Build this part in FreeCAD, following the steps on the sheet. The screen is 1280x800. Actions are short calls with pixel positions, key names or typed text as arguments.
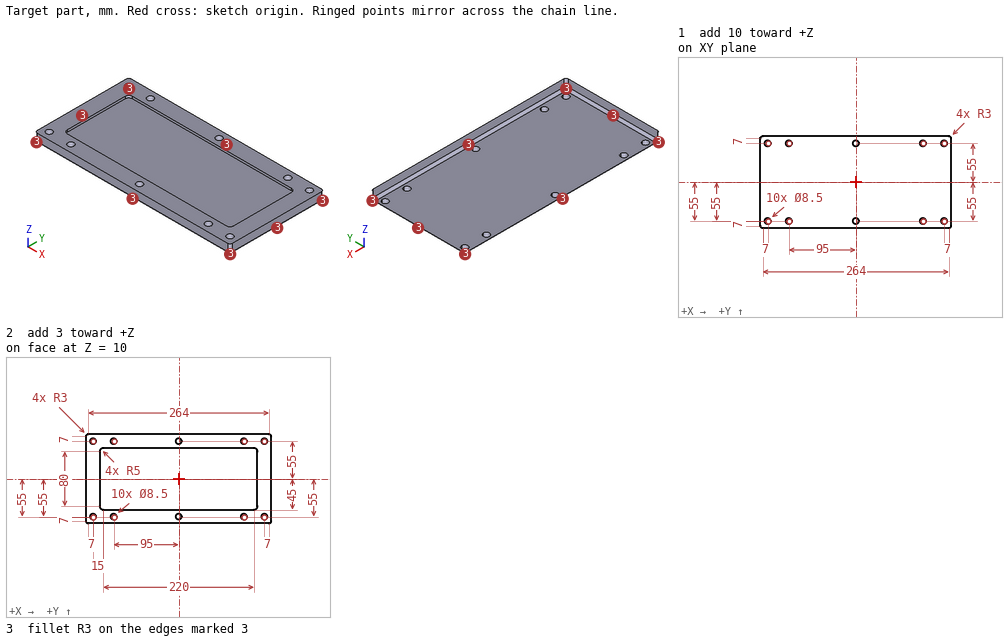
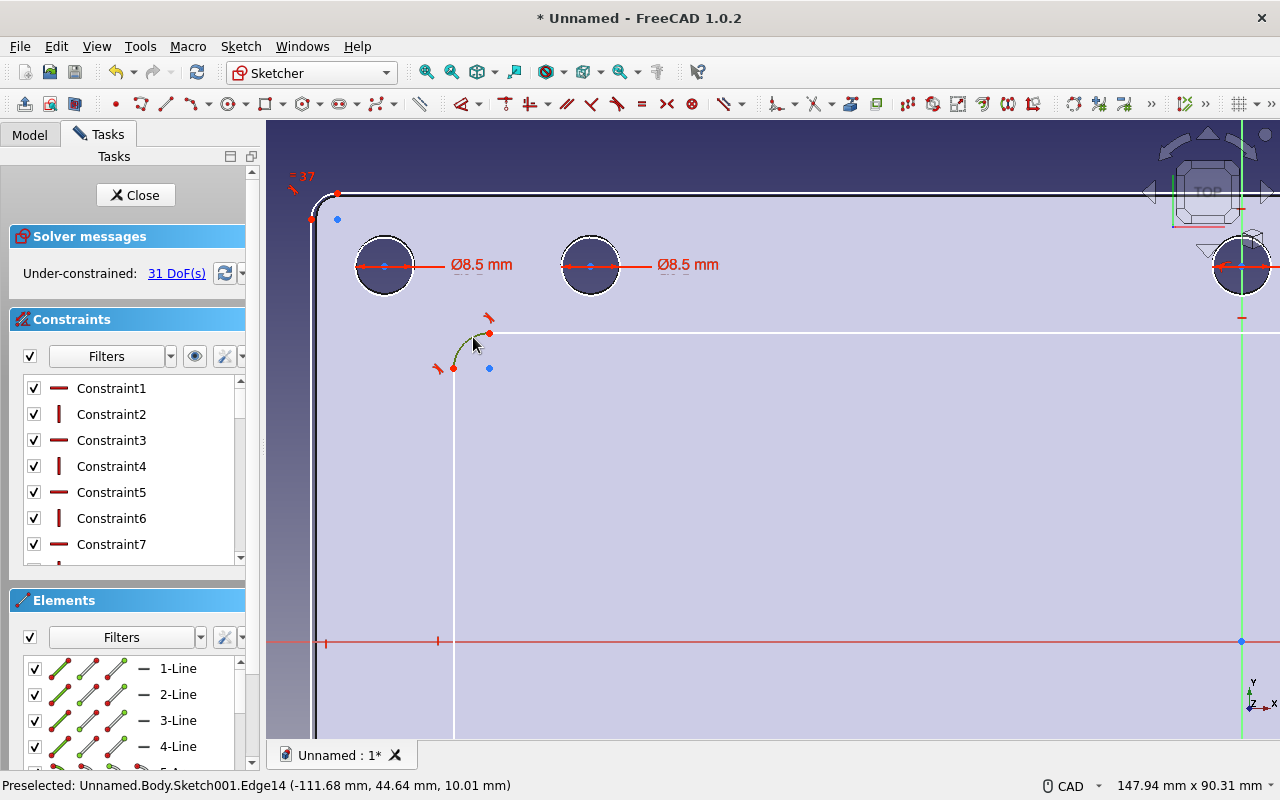
scroll(473, 338, down, 6)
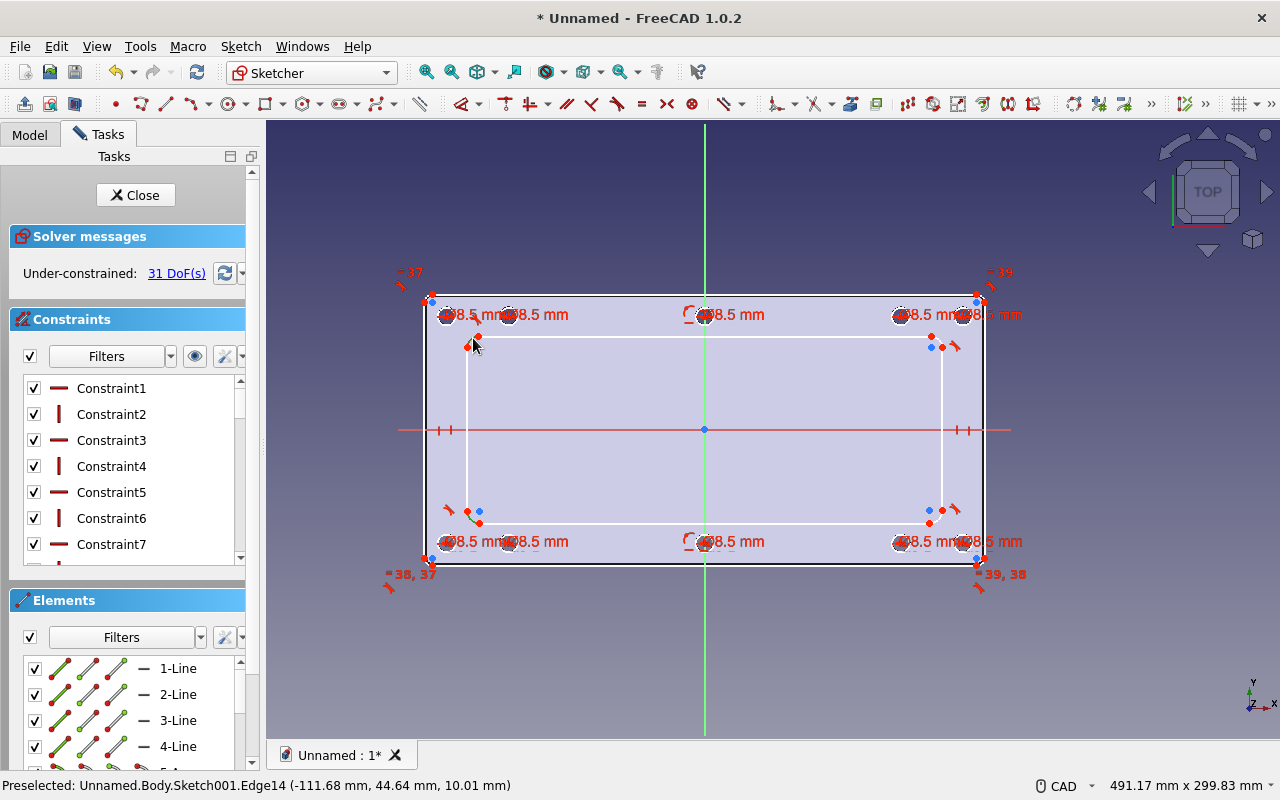
scroll(941, 343, up, 5)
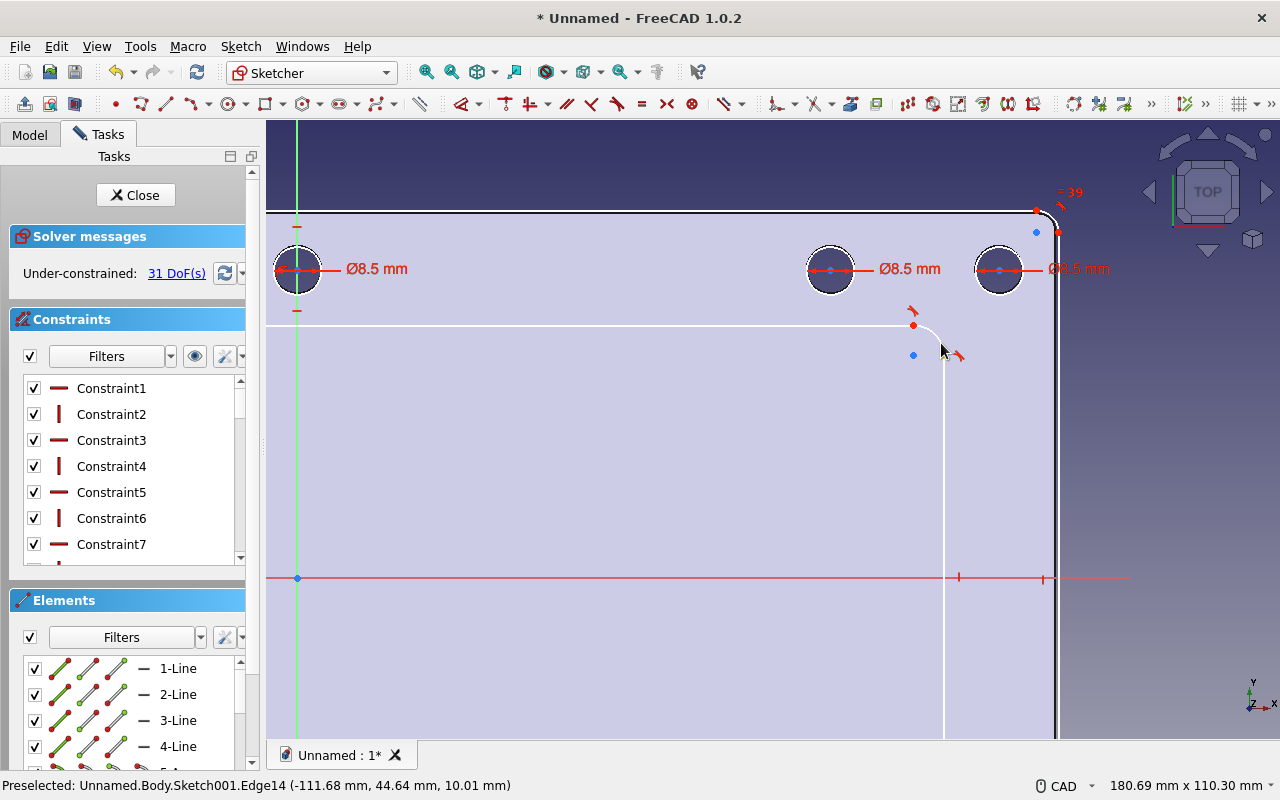
click(940, 342)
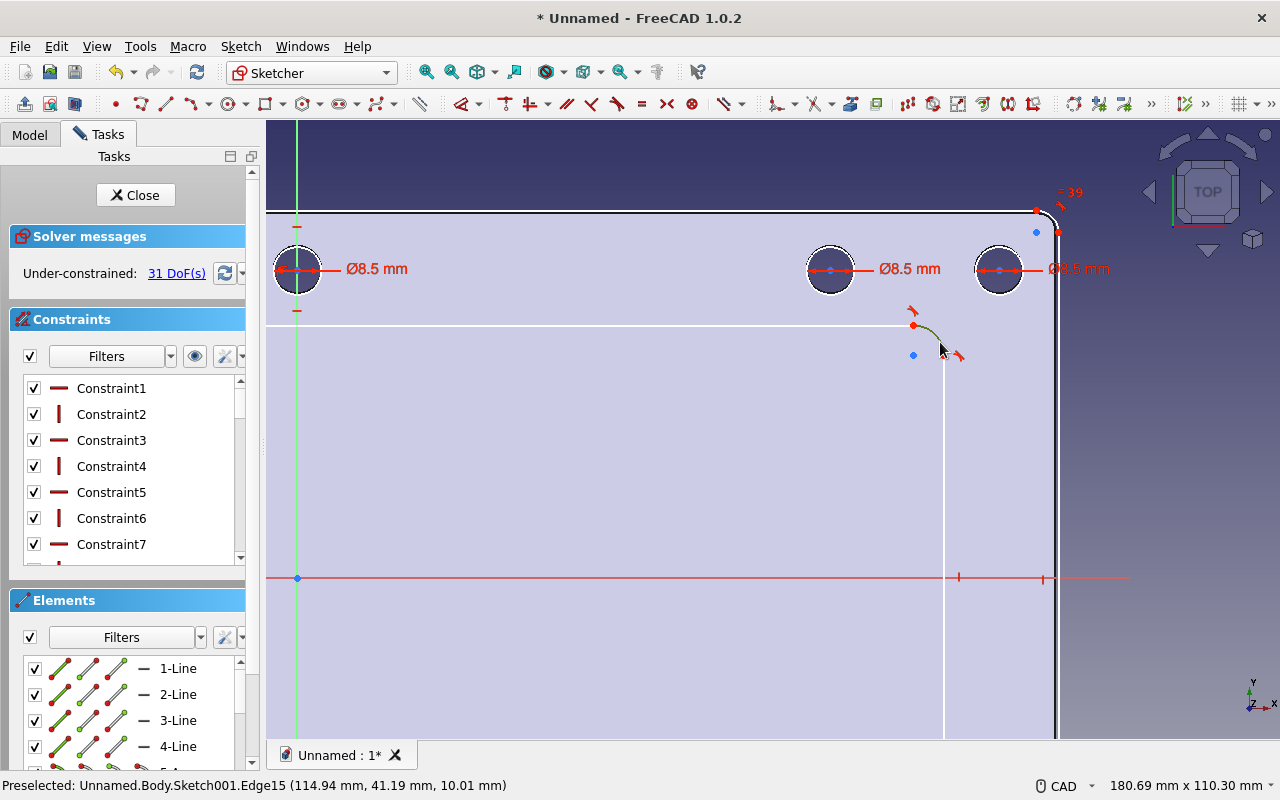
scroll(941, 343, down, 5)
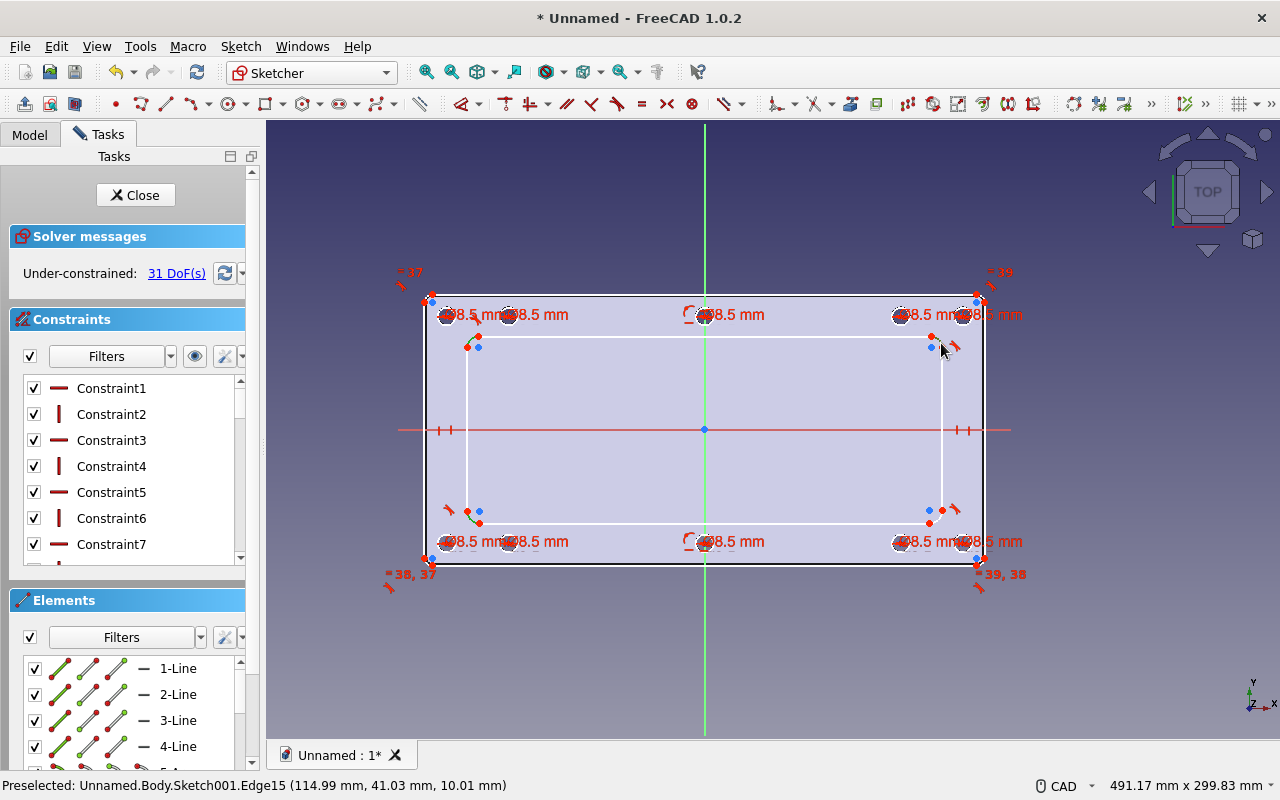
scroll(935, 522, up, 5)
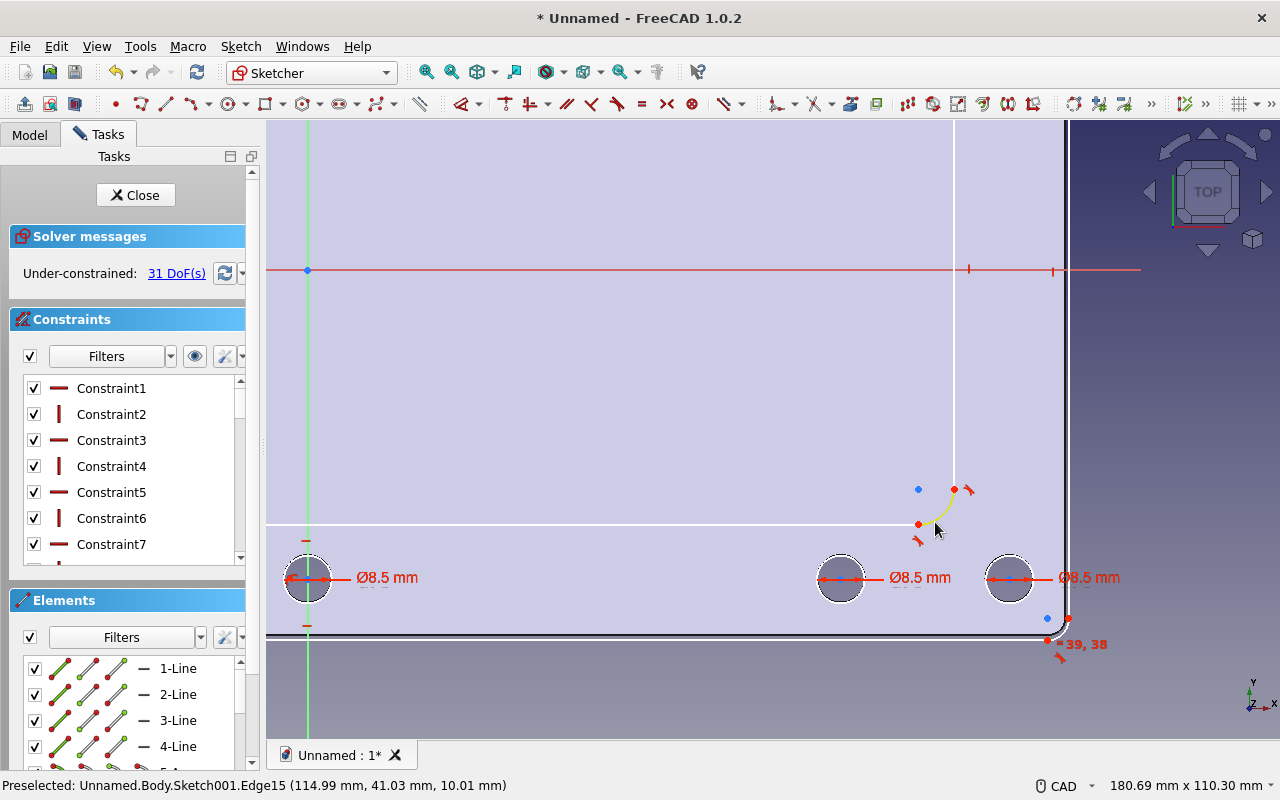
click(934, 521)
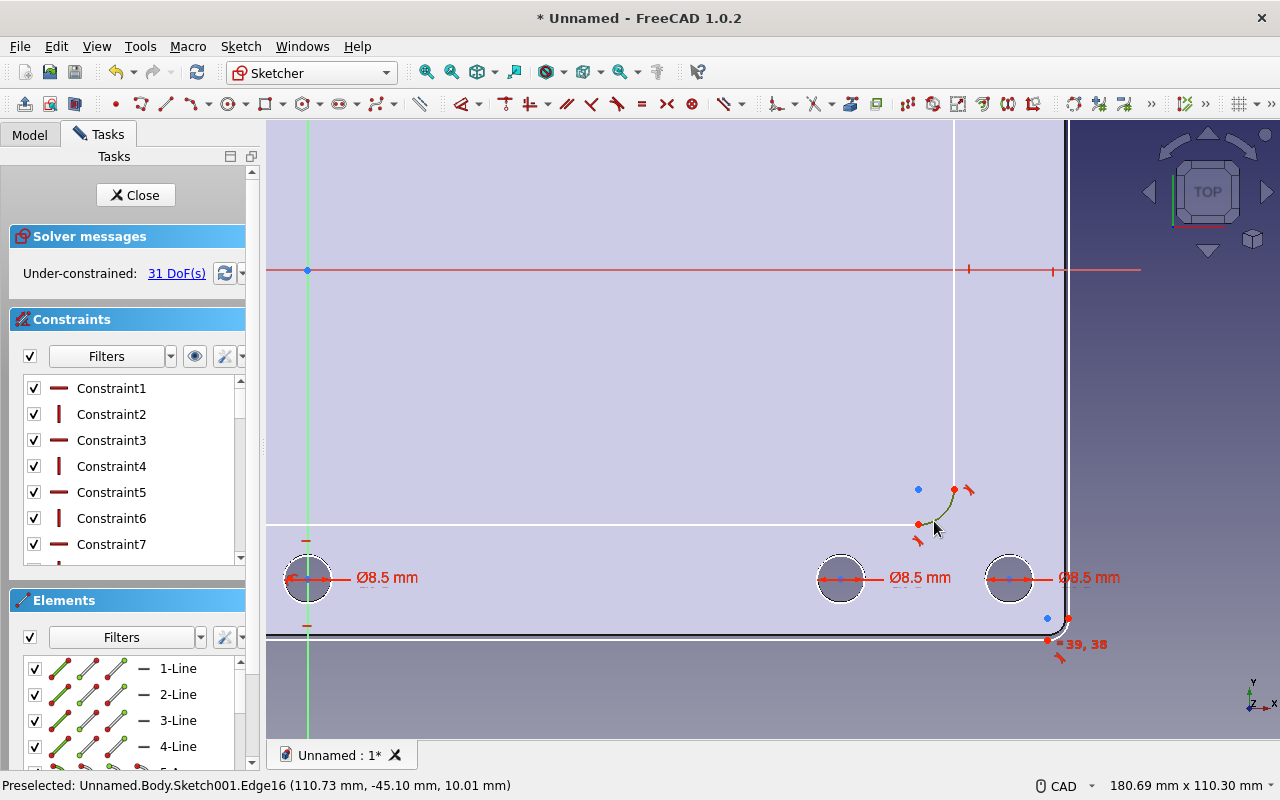
click(642, 104)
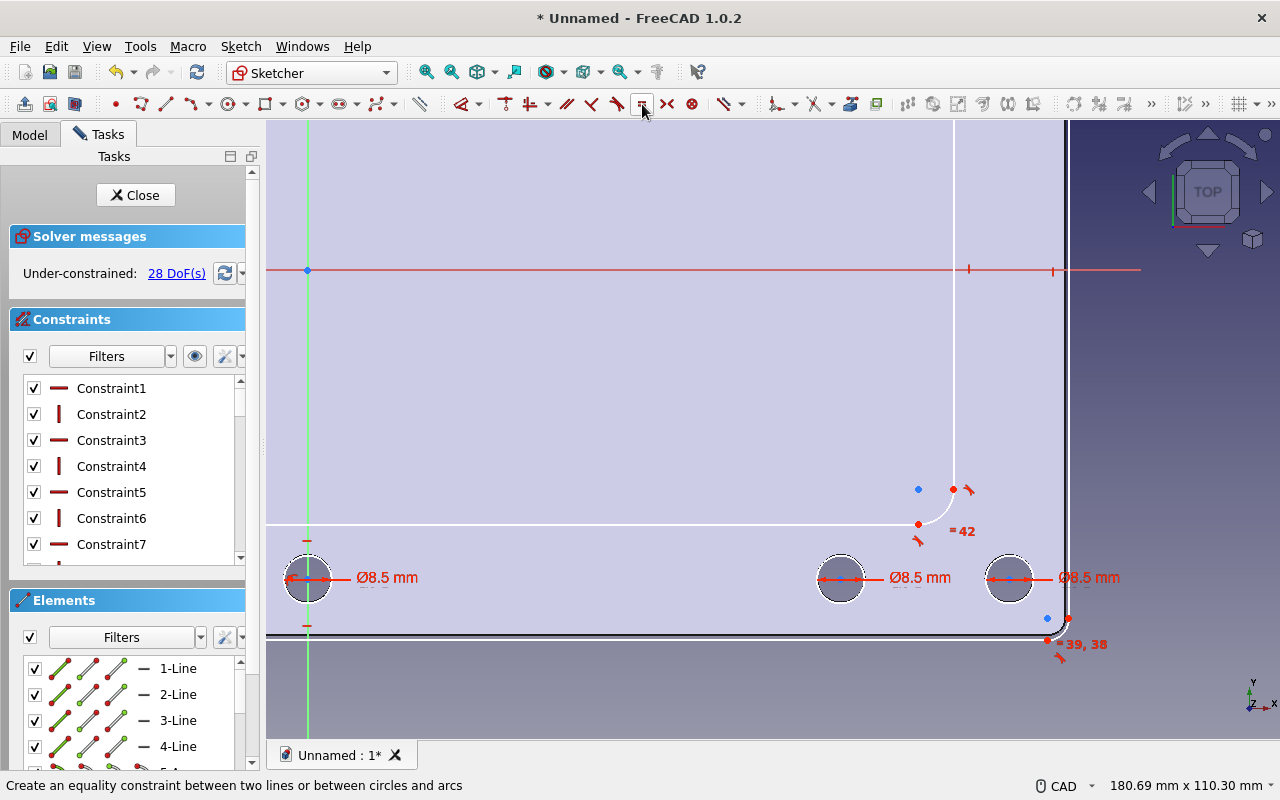
scroll(935, 522, down, 5)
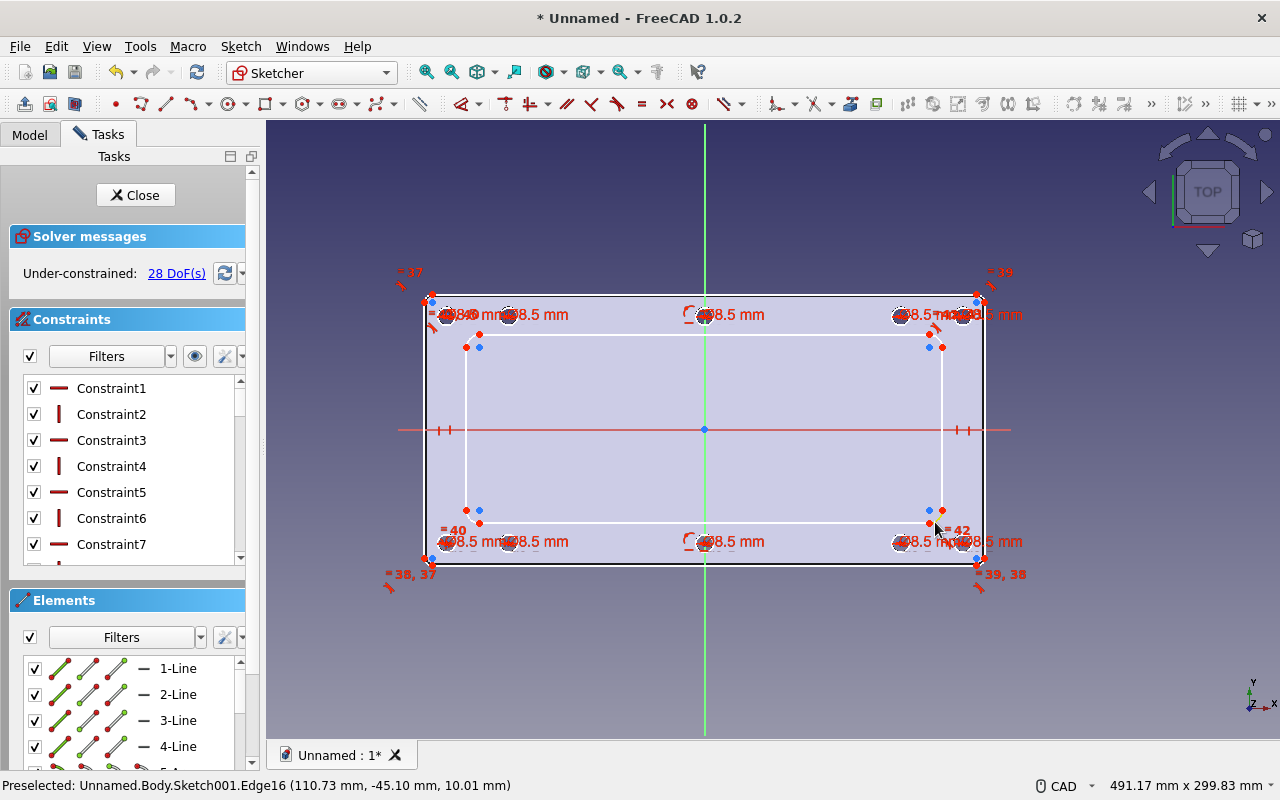
click(509, 544)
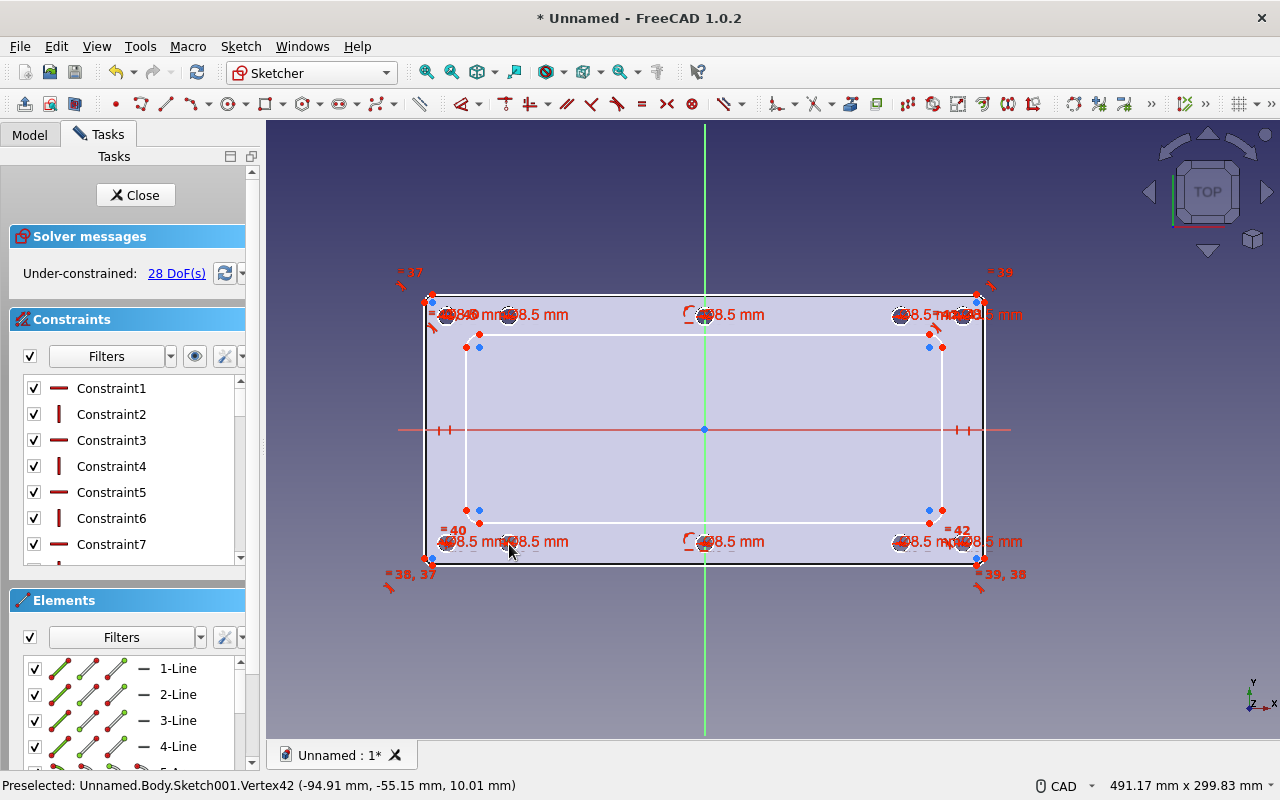
click(901, 544)